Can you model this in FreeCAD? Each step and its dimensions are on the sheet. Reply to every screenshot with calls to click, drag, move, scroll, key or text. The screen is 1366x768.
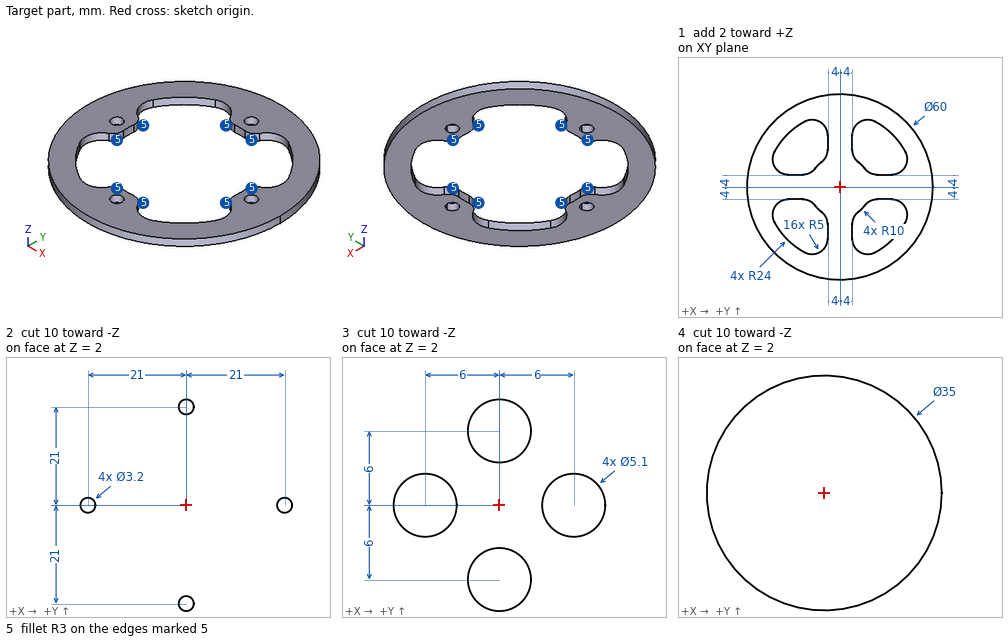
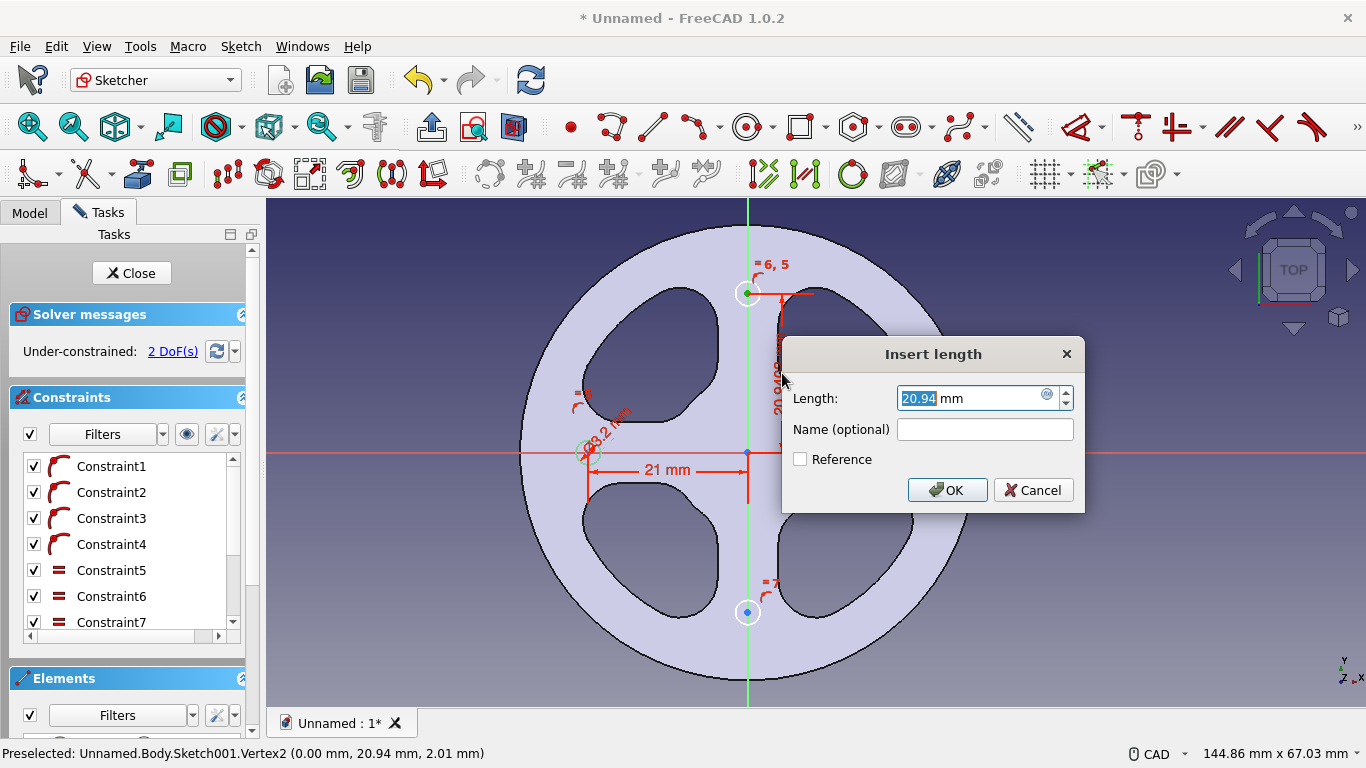
text(21)
key(Return)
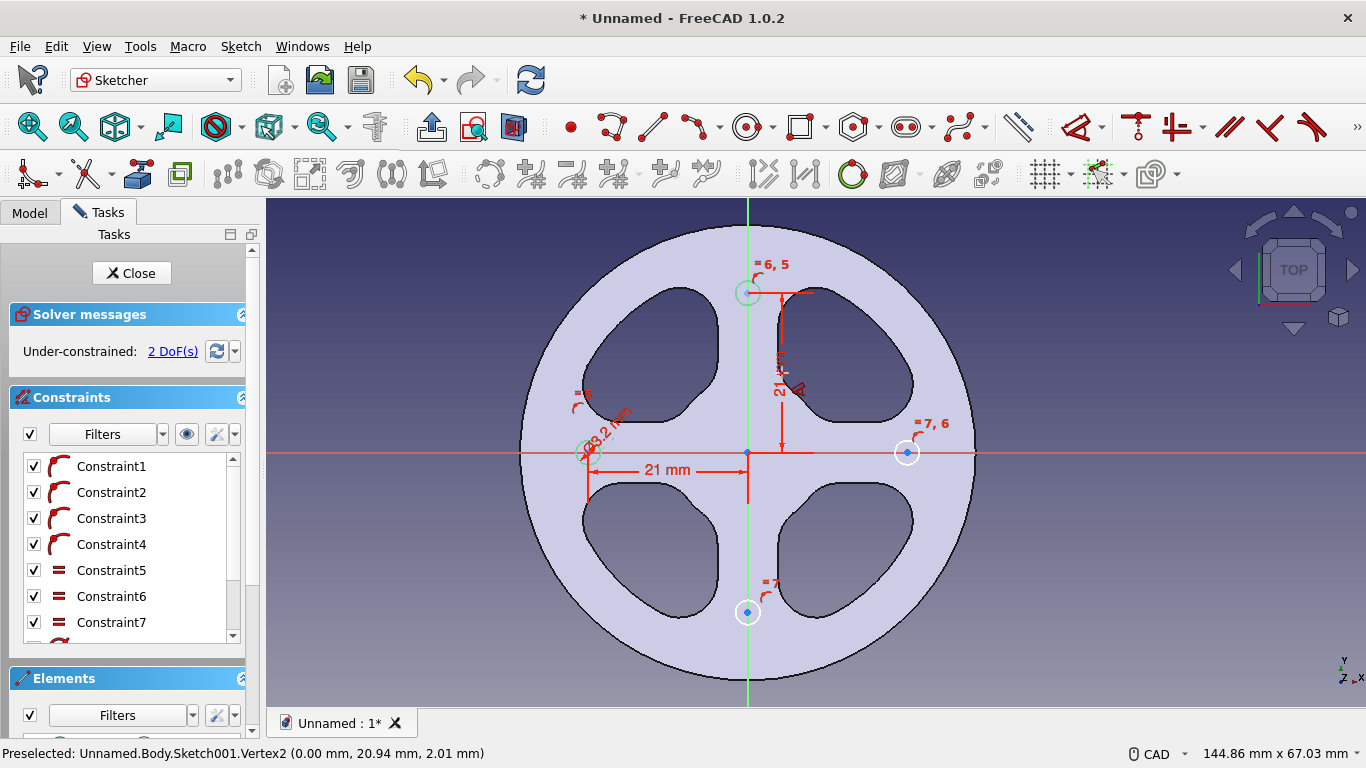
click(907, 453)
click(828, 487)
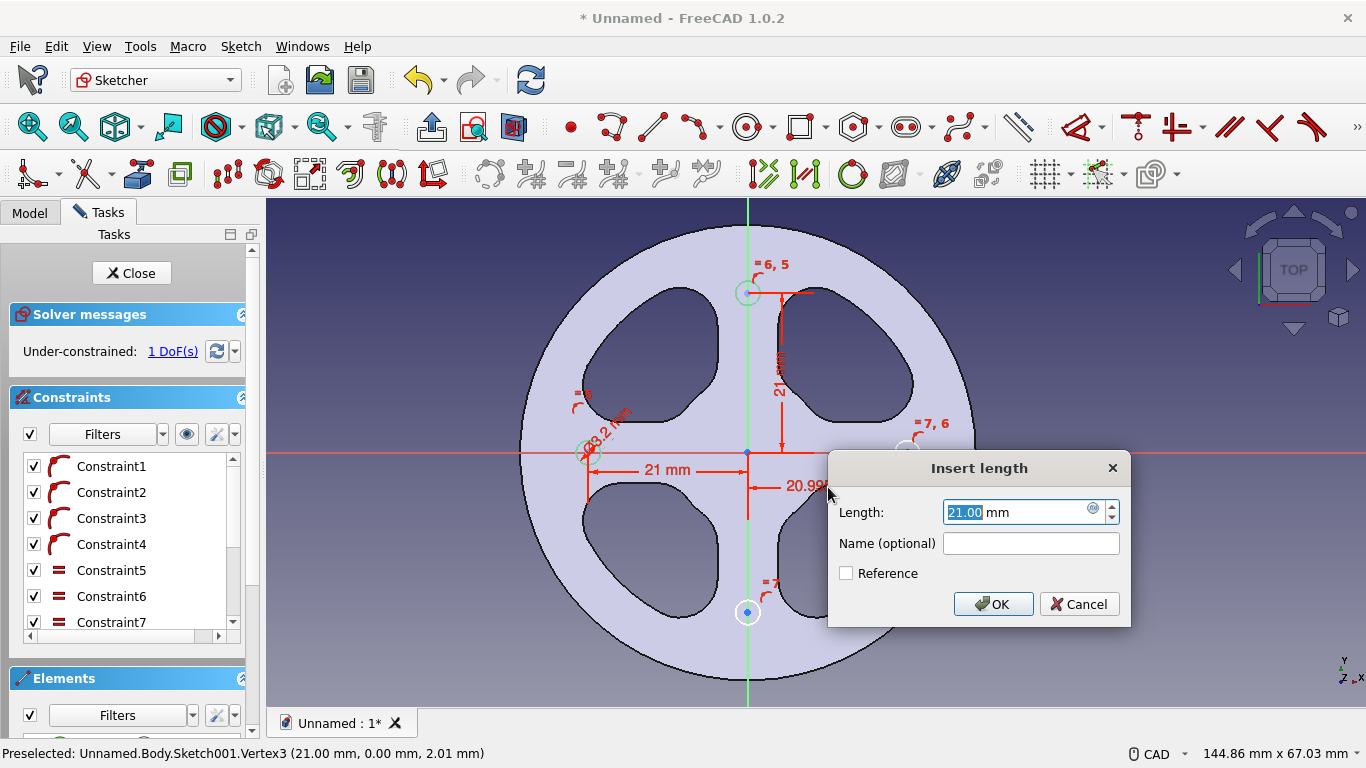
text(21)
key(Return)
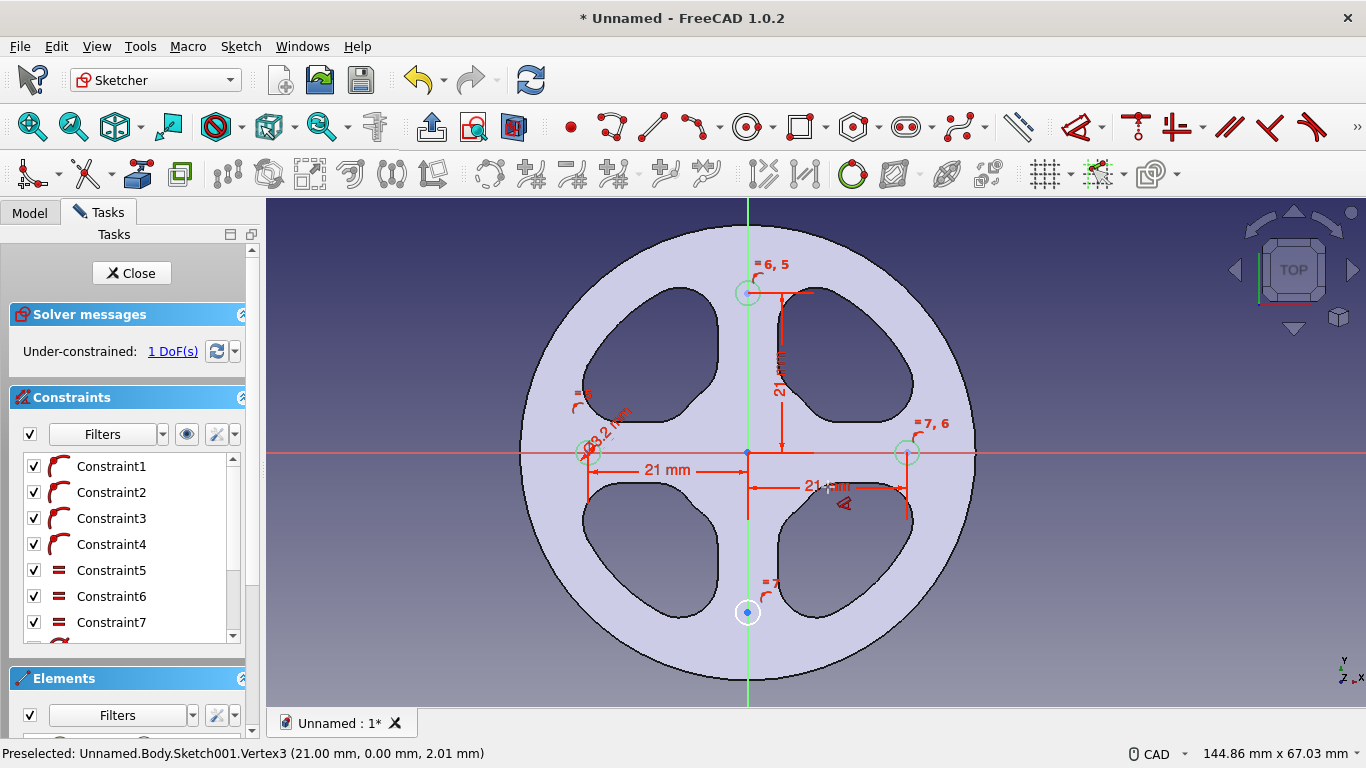
click(748, 613)
click(782, 533)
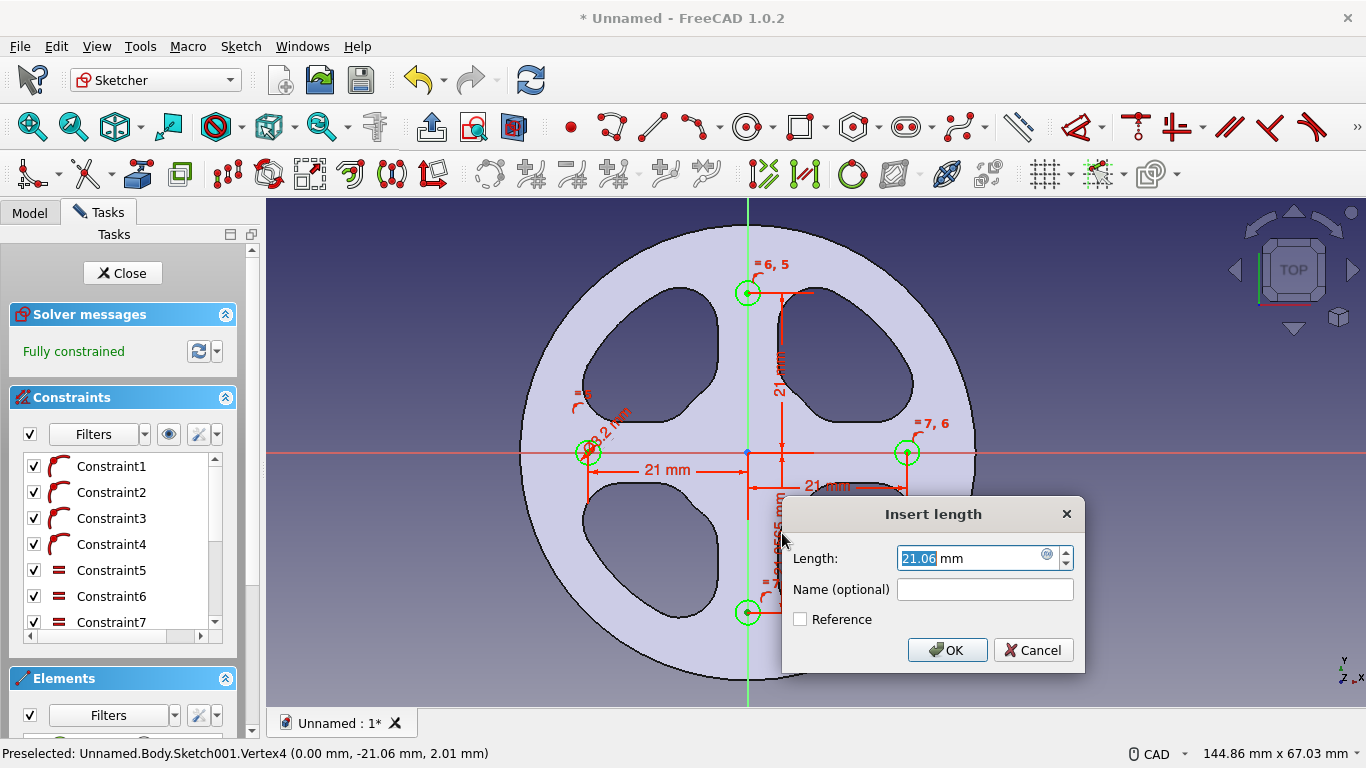
text(21)
key(Return)
key(Escape)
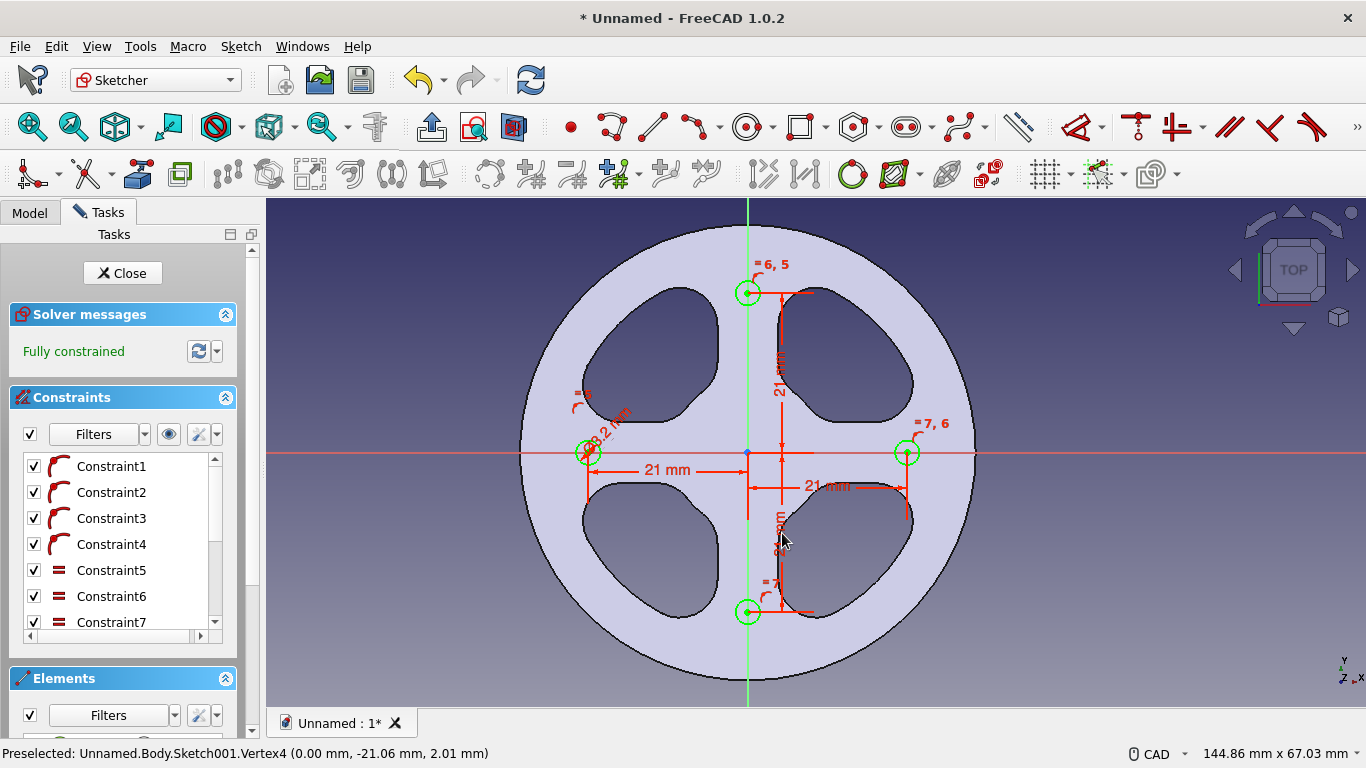
click(123, 273)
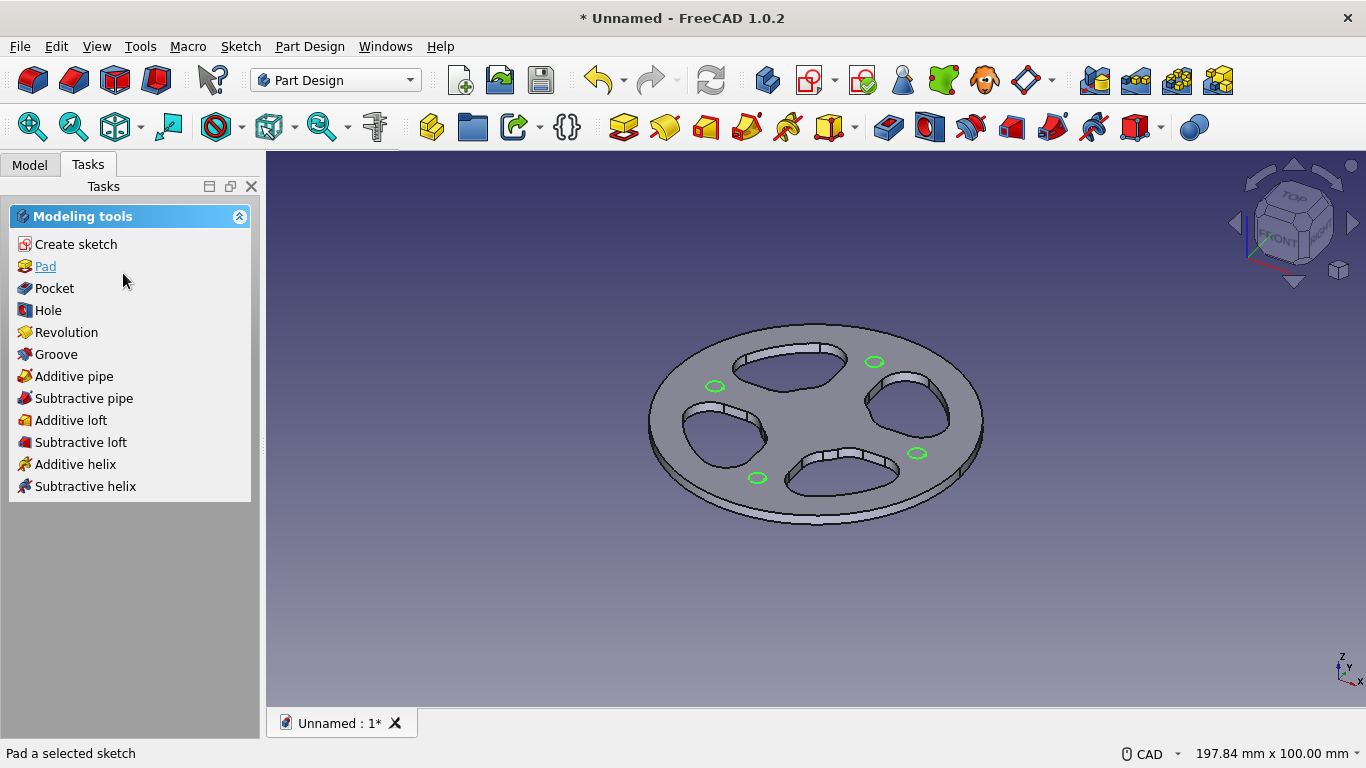
click(889, 128)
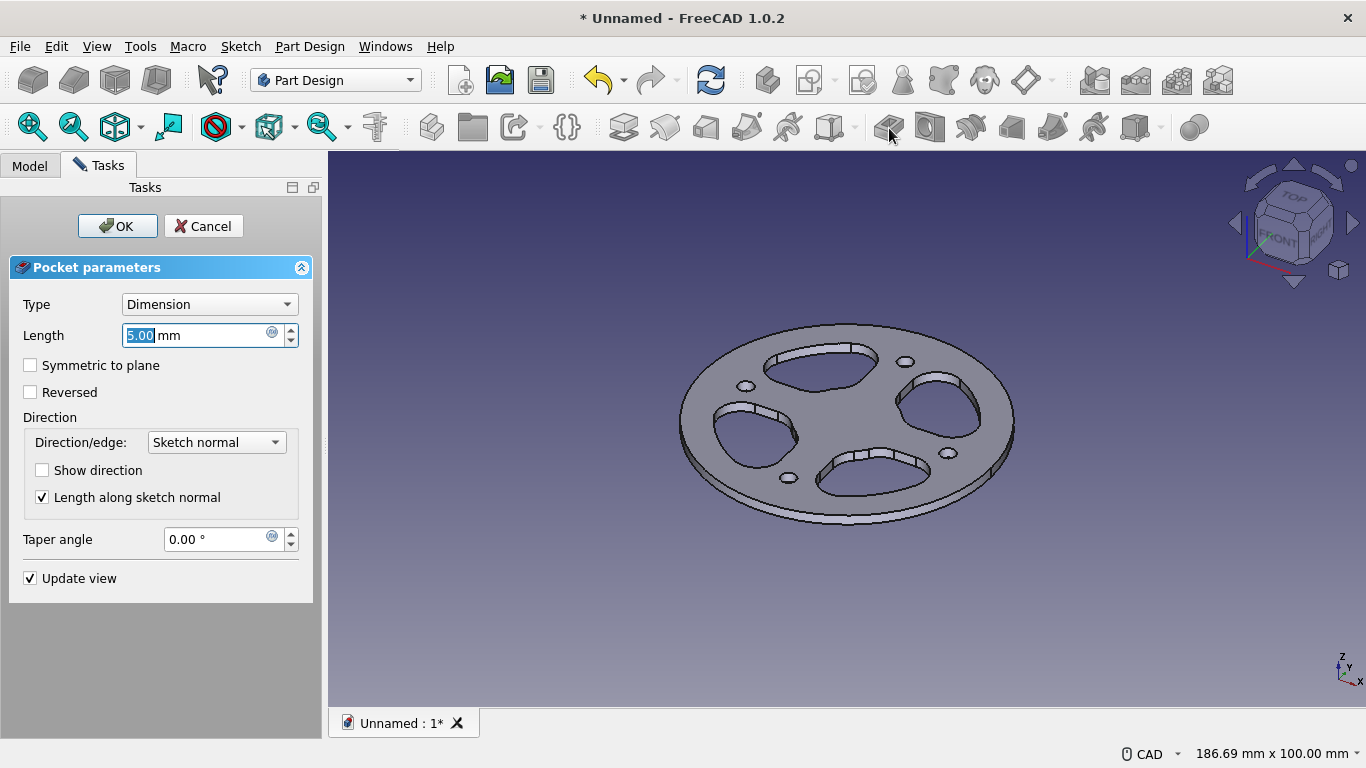
text(10)
key(Tab)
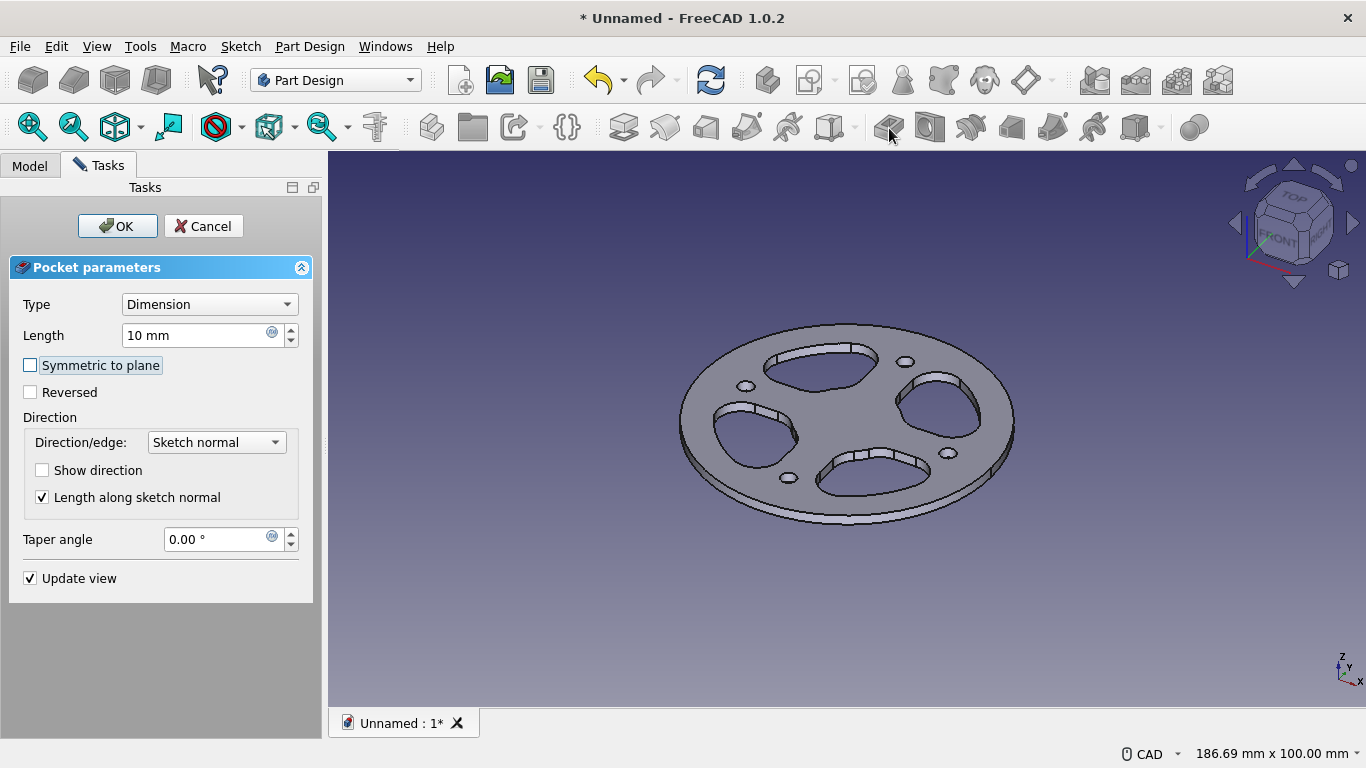
click(118, 226)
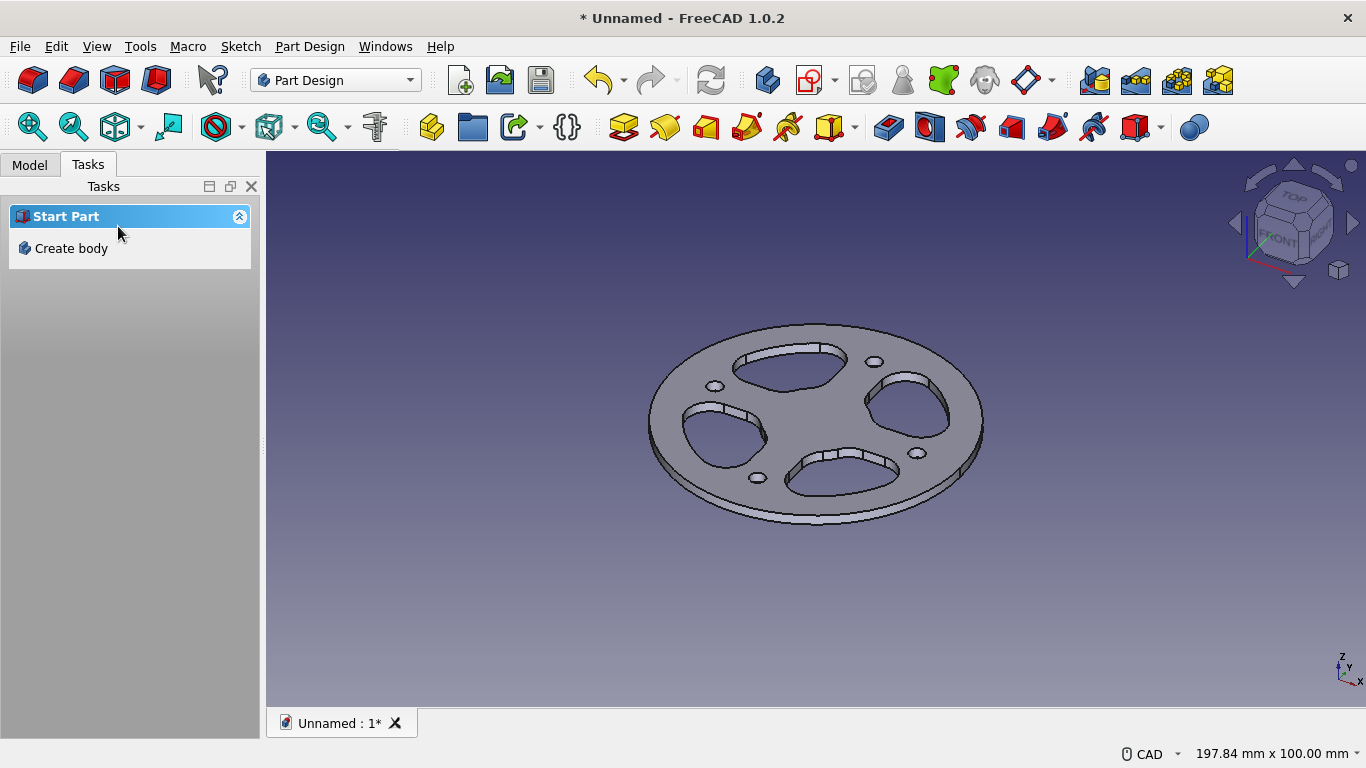
click(816, 419)